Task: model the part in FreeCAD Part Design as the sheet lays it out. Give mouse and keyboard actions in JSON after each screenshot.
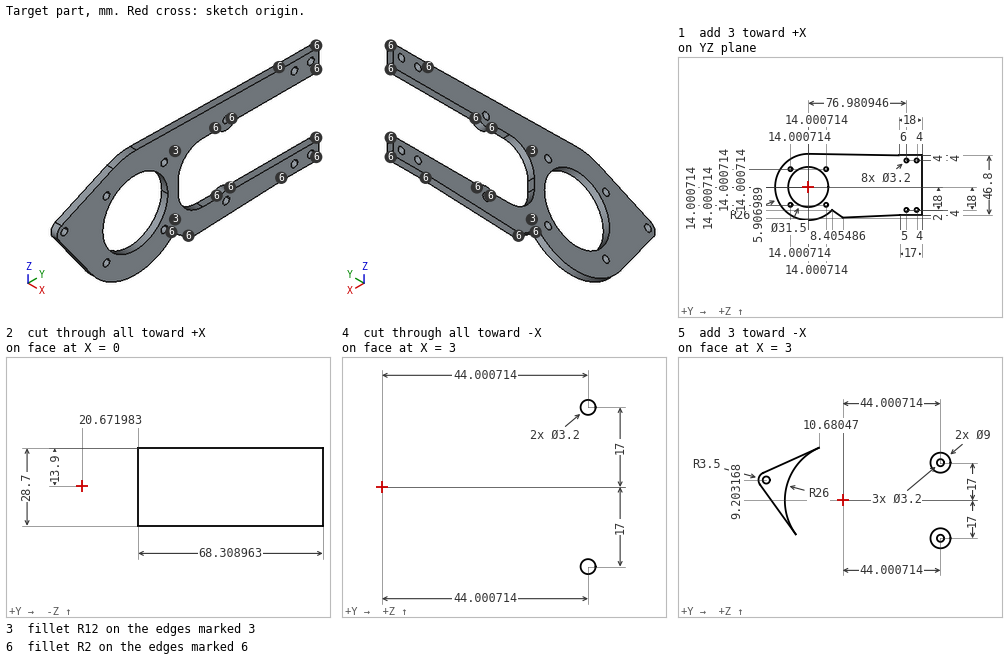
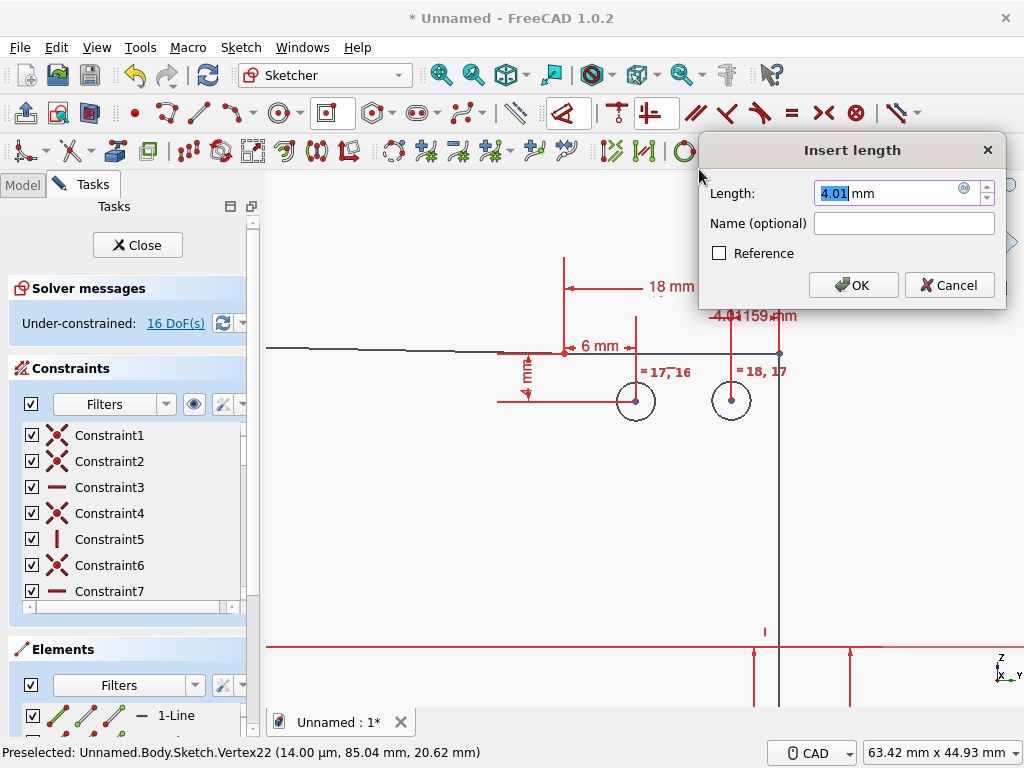
{"action": "type", "text": "4"}
{"action": "key", "text": "Return"}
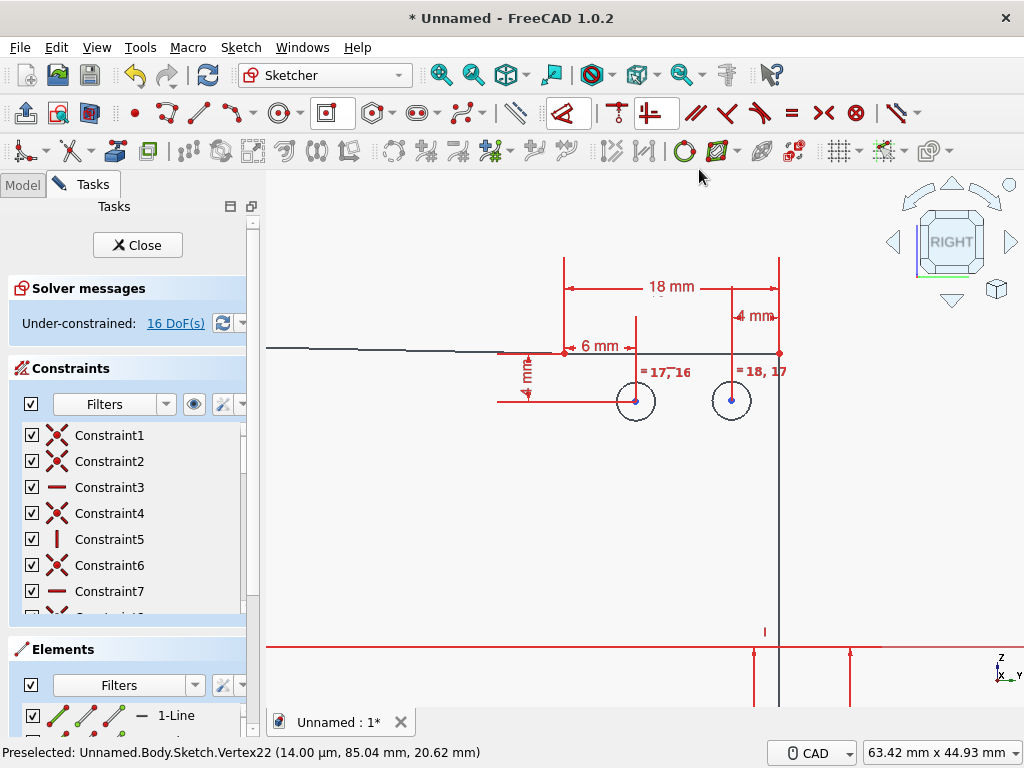
{"action": "left_click", "coordinate": [779, 354]}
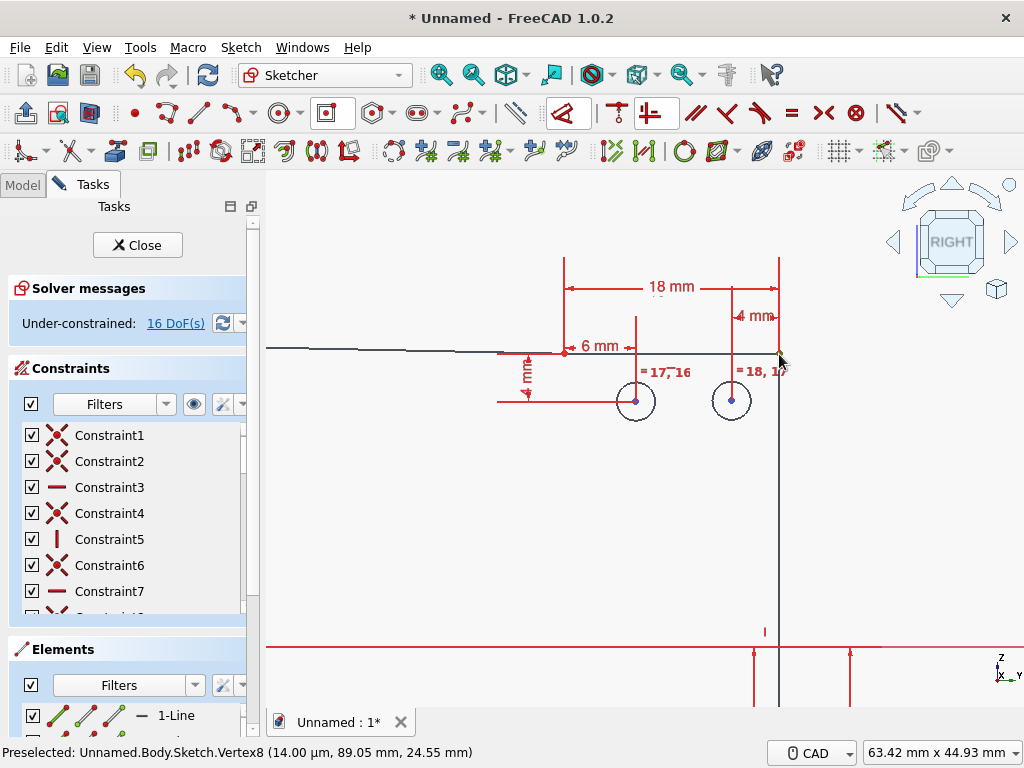
{"action": "left_click", "coordinate": [732, 401]}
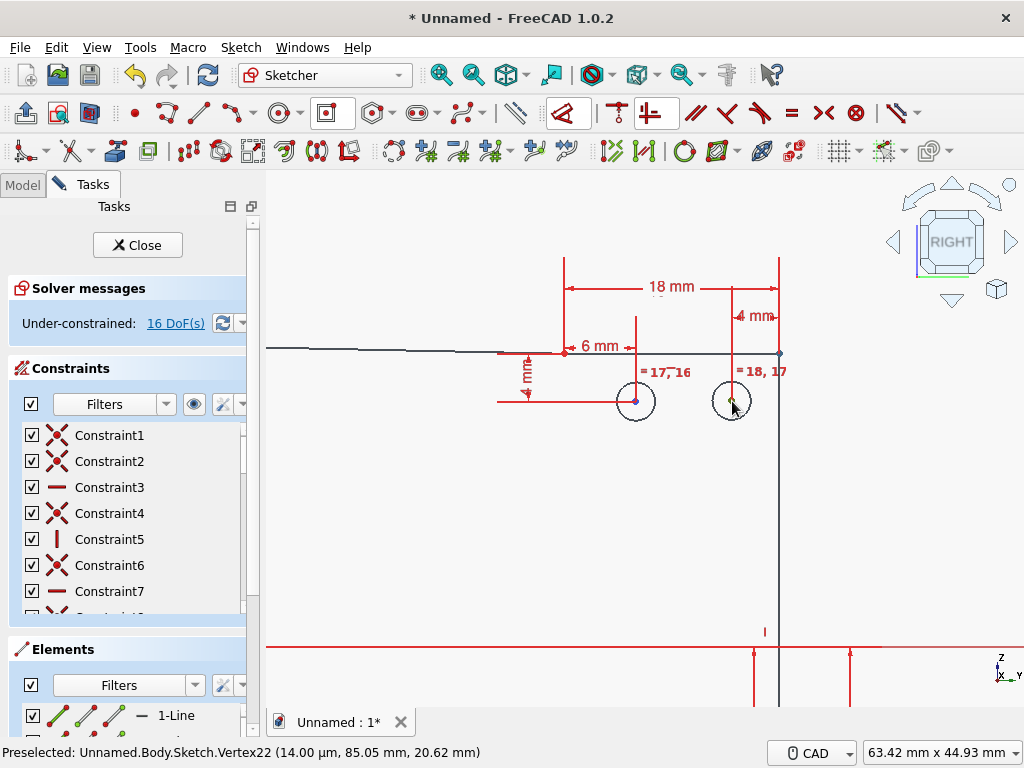
{"action": "key", "text": "i"}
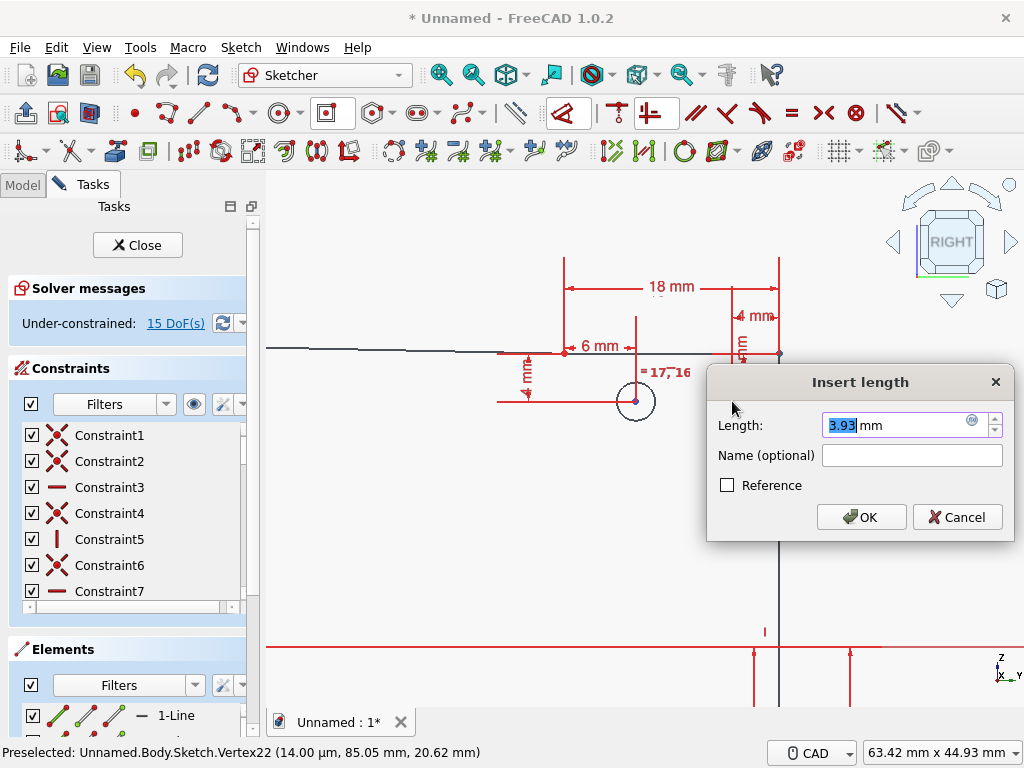
{"action": "type", "text": "4"}
{"action": "key", "text": "Return"}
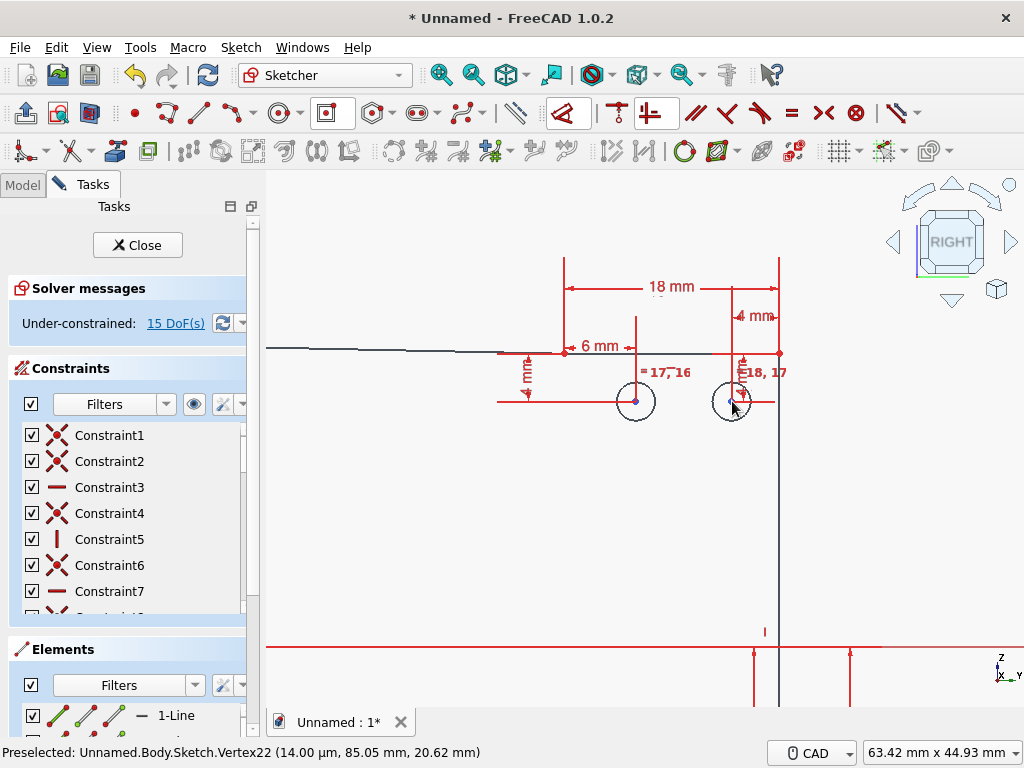
{"action": "scroll", "coordinate": [780, 354], "scroll_direction": "down", "scroll_amount": 6}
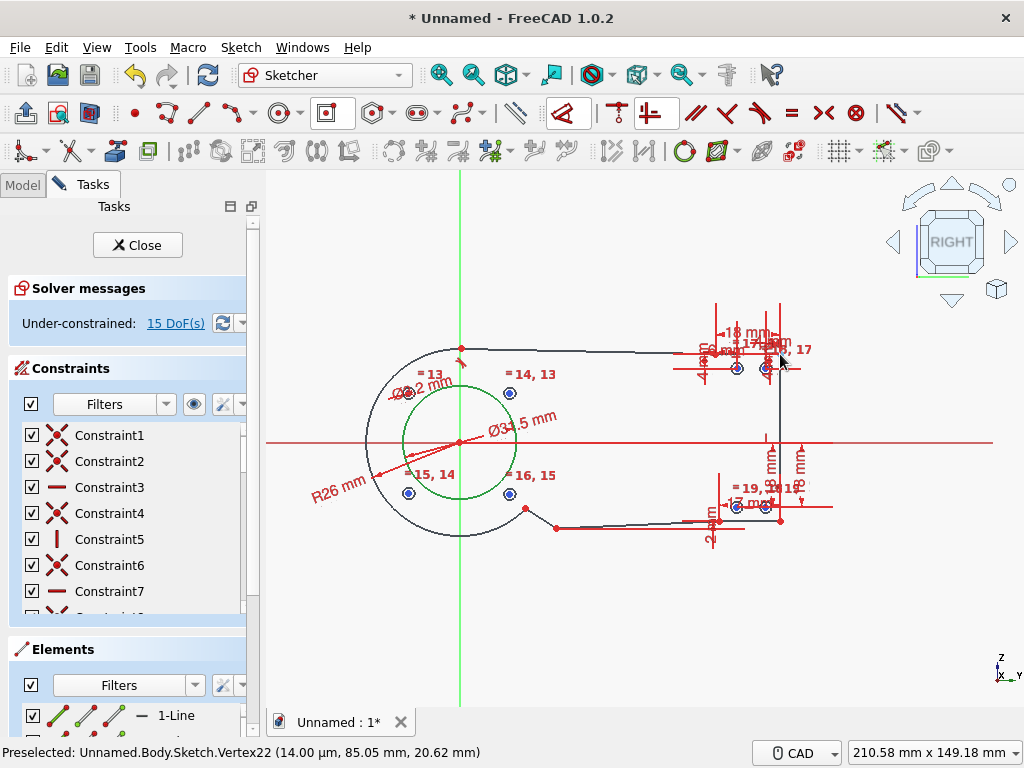
{"action": "scroll", "coordinate": [719, 521], "scroll_direction": "up", "scroll_amount": 4}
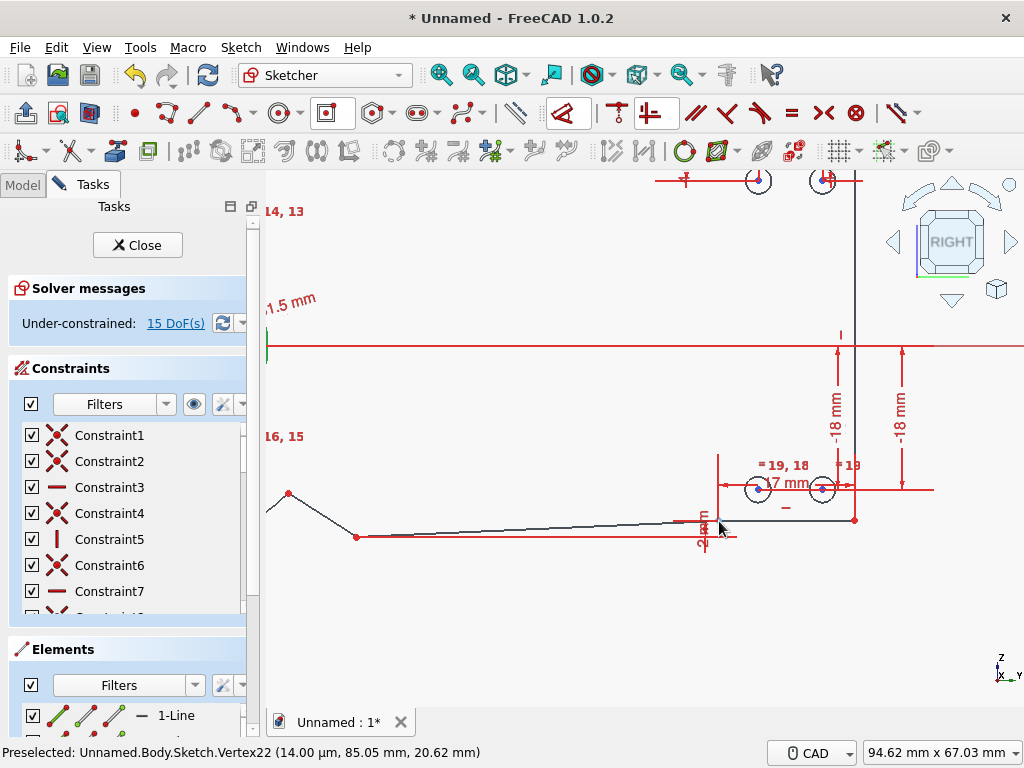
{"action": "left_click", "coordinate": [718, 521]}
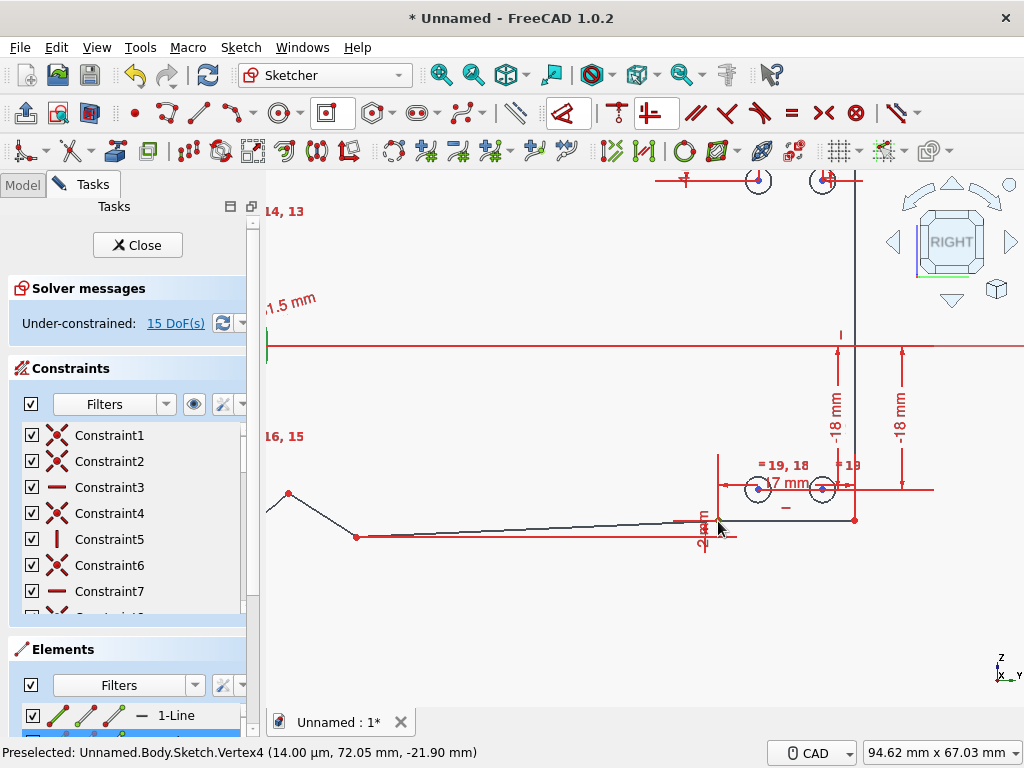
{"action": "left_click", "coordinate": [758, 490]}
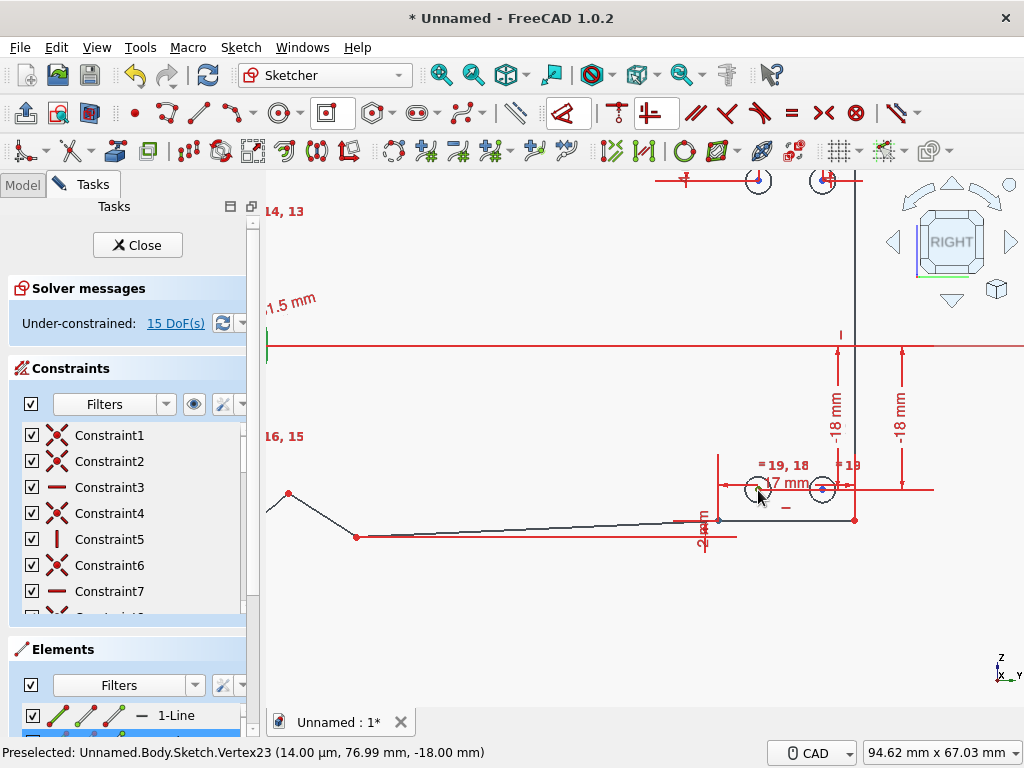
{"action": "left_click", "coordinate": [586, 114]}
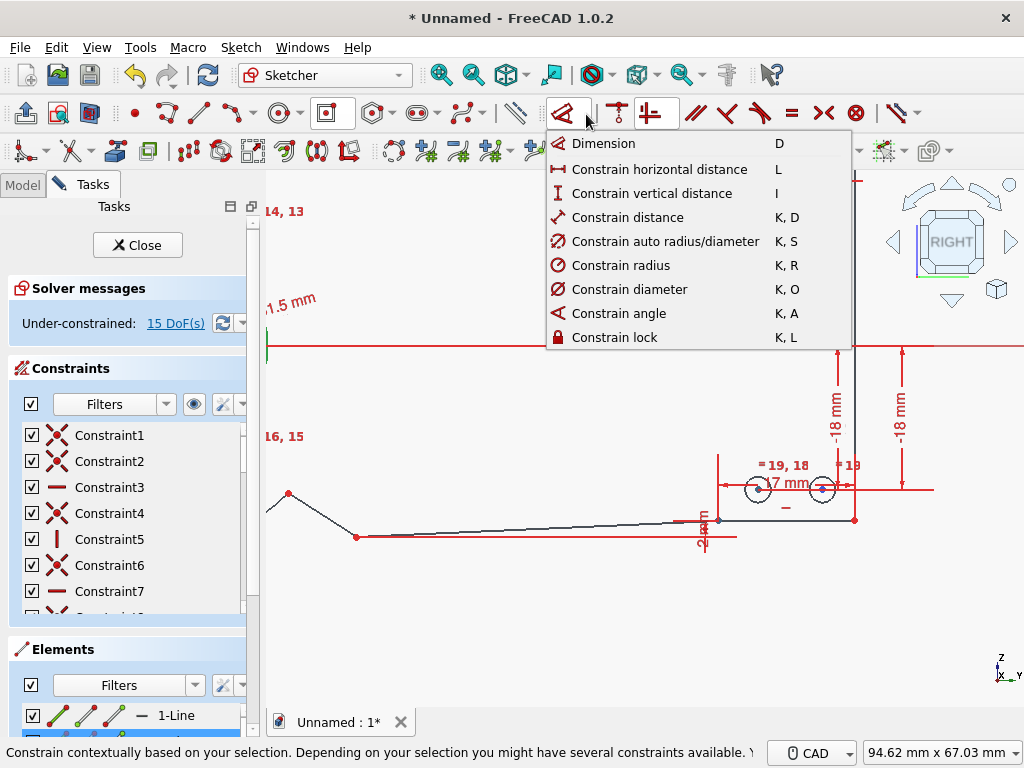
{"action": "left_click", "coordinate": [699, 169]}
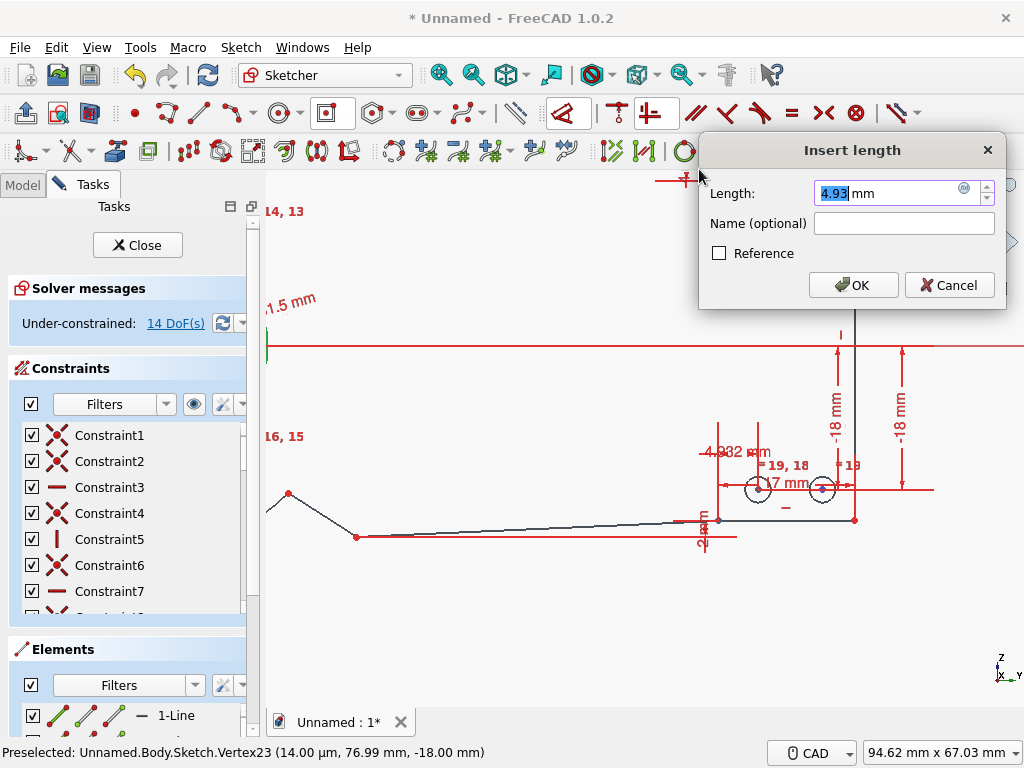
{"action": "type", "text": "5"}
{"action": "key", "text": "Return"}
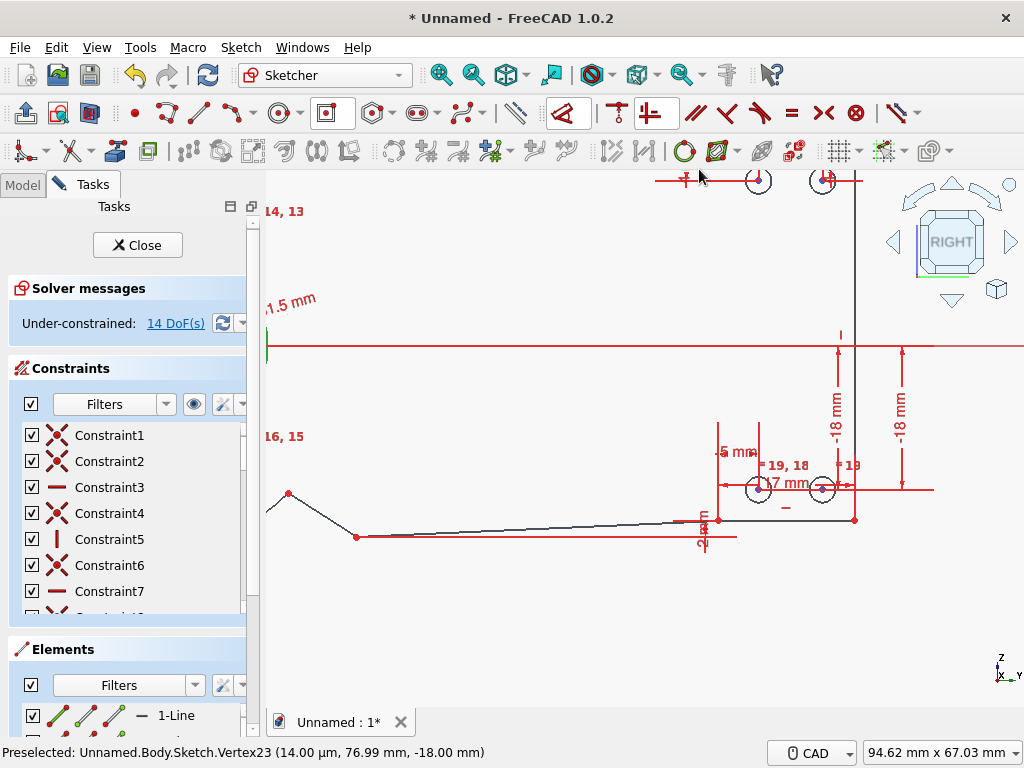
{"action": "scroll", "coordinate": [718, 521], "scroll_direction": "up", "scroll_amount": 2}